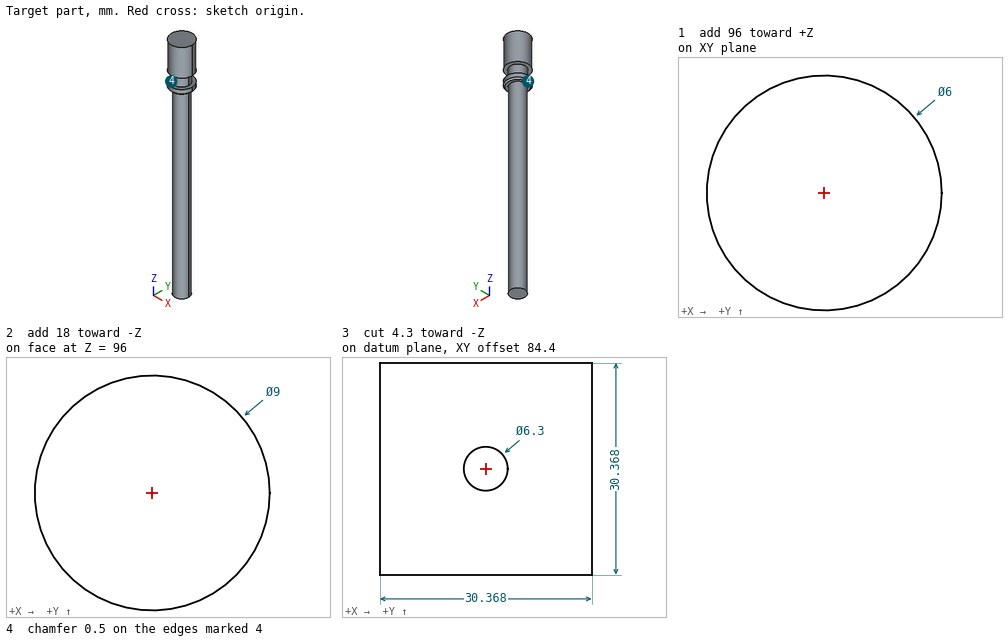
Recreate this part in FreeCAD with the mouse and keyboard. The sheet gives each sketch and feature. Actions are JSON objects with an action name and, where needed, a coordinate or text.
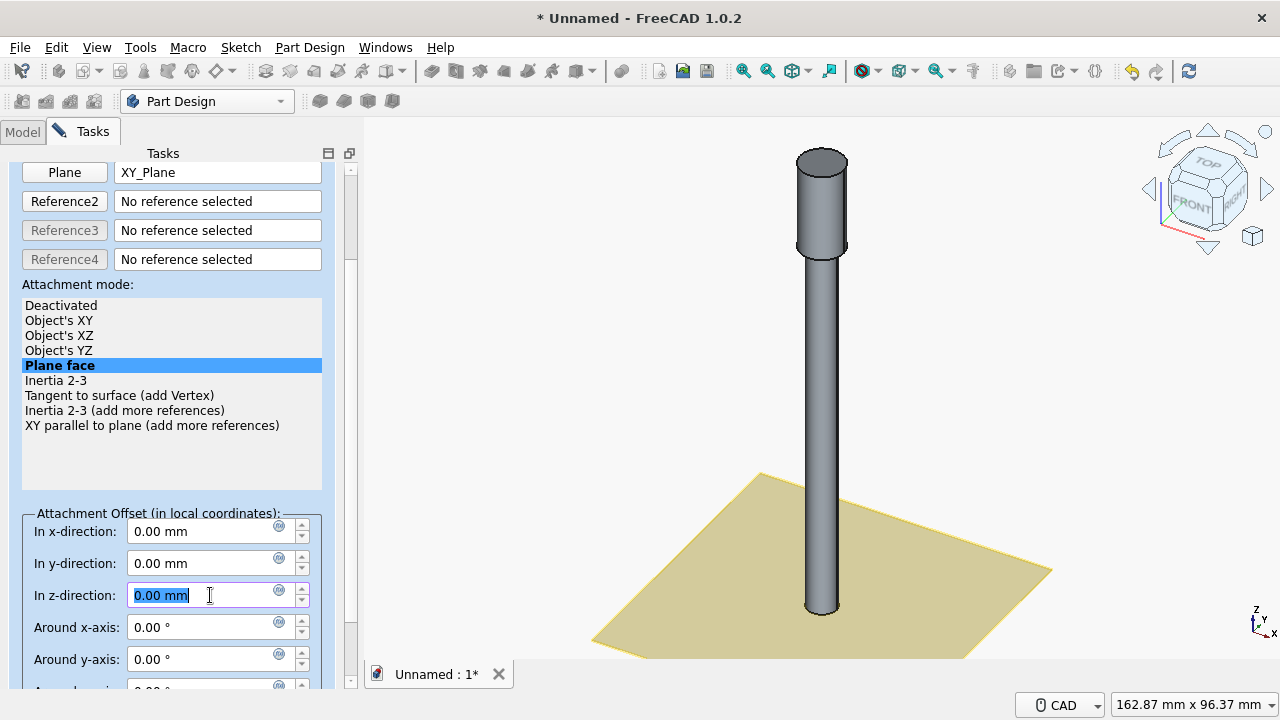
{"action": "type", "text": "84.4"}
{"action": "key", "text": "Tab"}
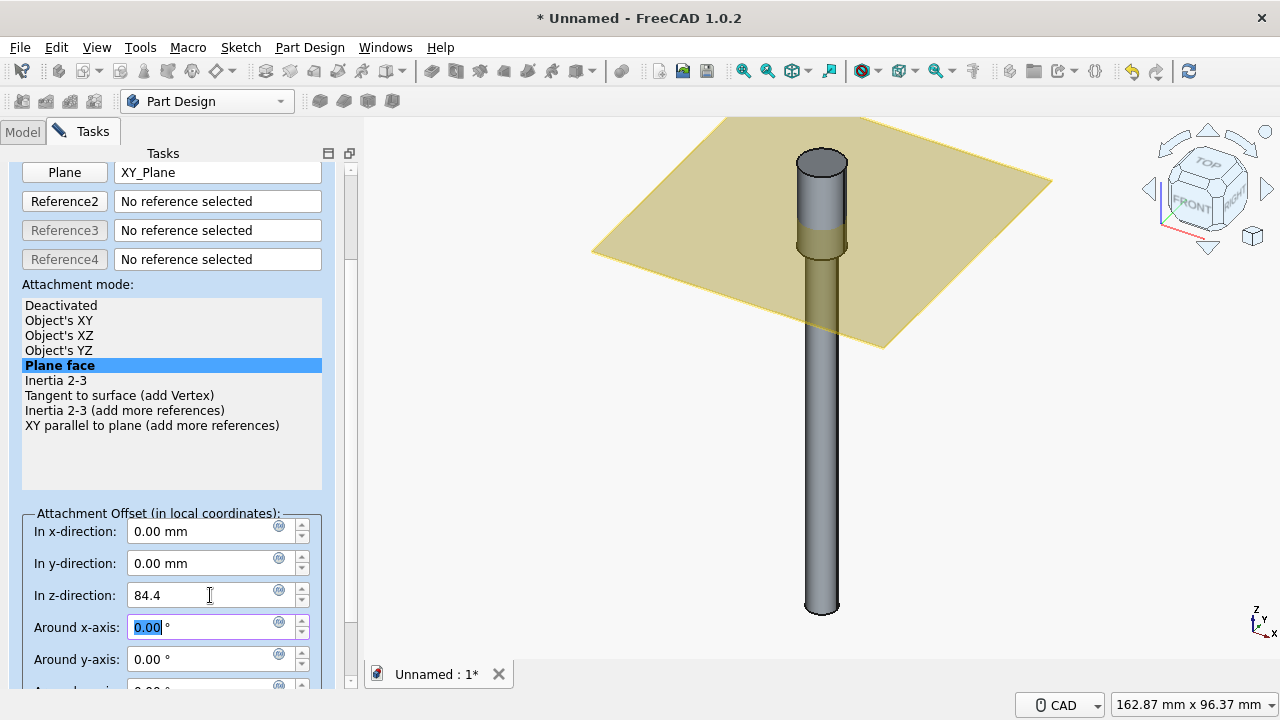
{"action": "scroll", "coordinate": [351, 426], "scroll_direction": "up", "scroll_amount": 3}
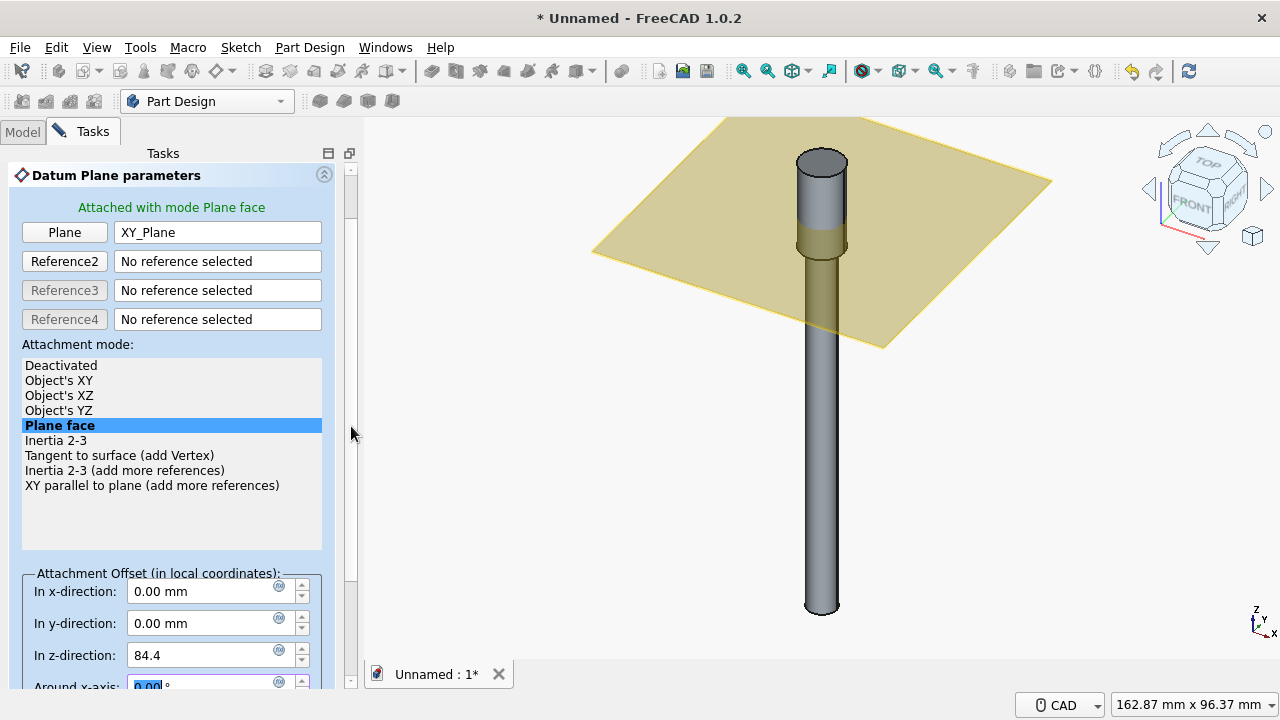
{"action": "left_click", "coordinate": [124, 192]}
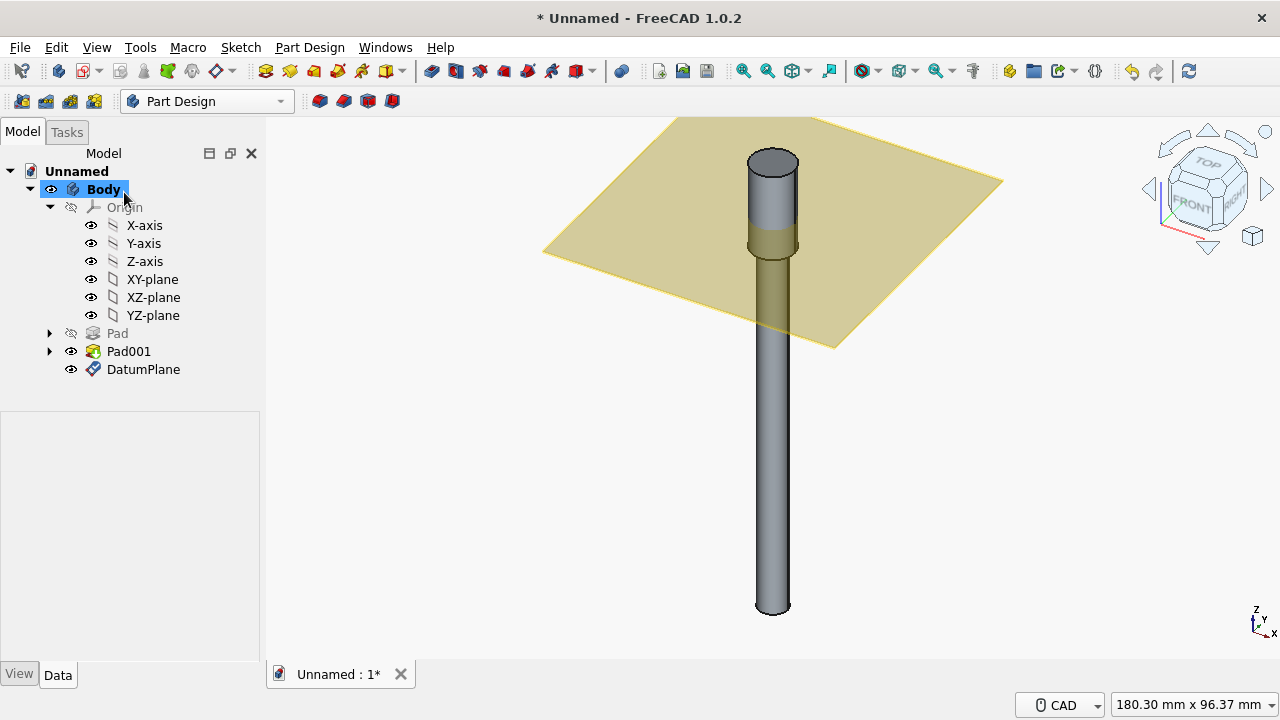
{"action": "left_click", "coordinate": [116, 369]}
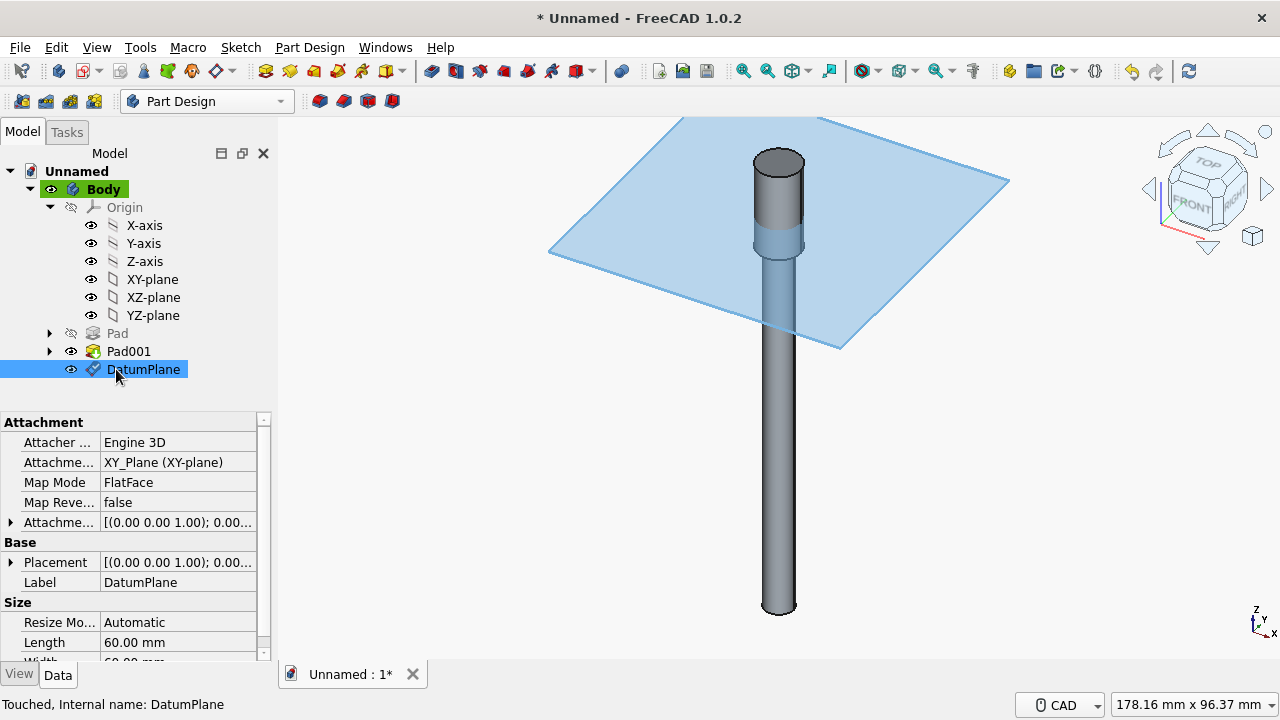
{"action": "left_click", "coordinate": [84, 72]}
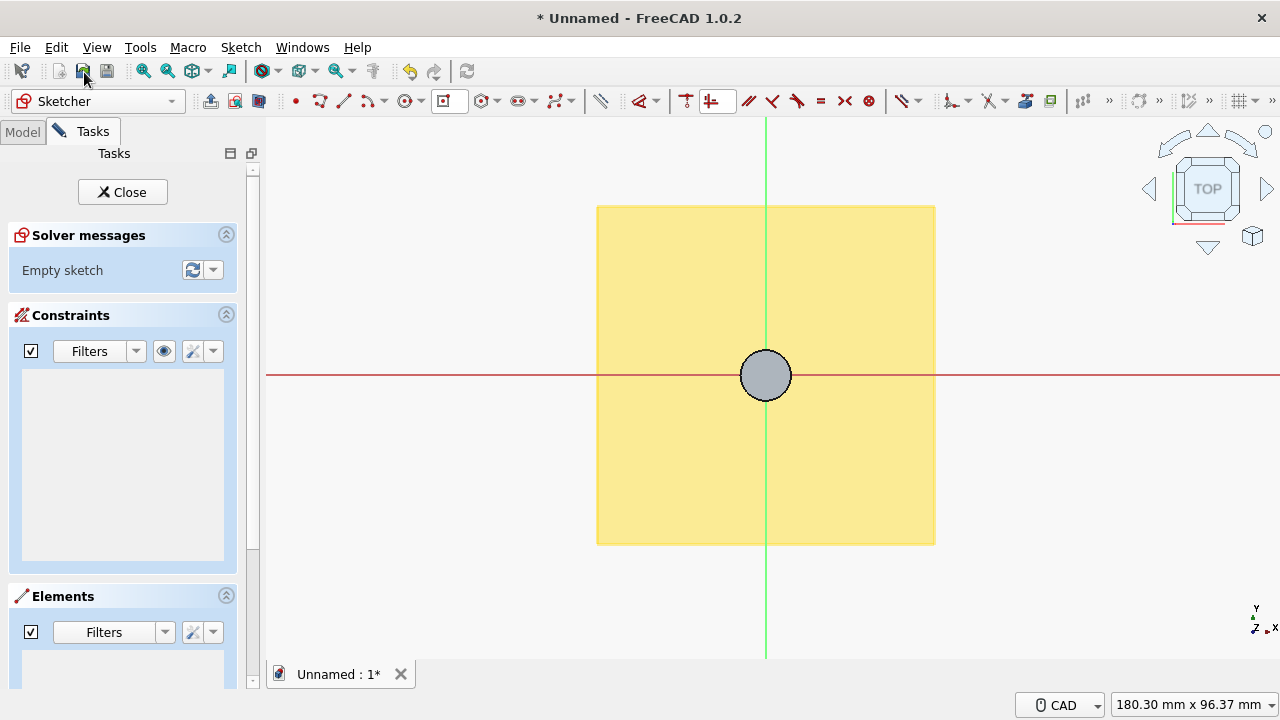
{"action": "left_click", "coordinate": [260, 102]}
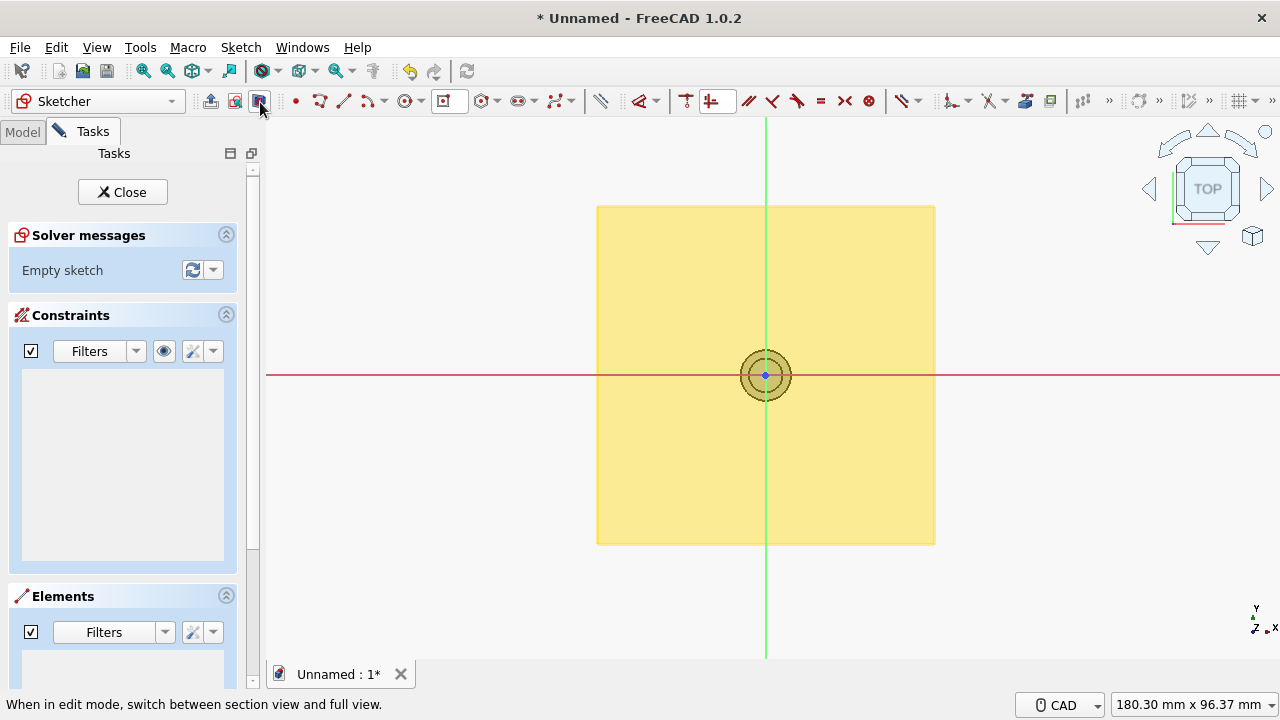
{"action": "scroll", "coordinate": [840, 360], "scroll_direction": "up", "scroll_amount": 3}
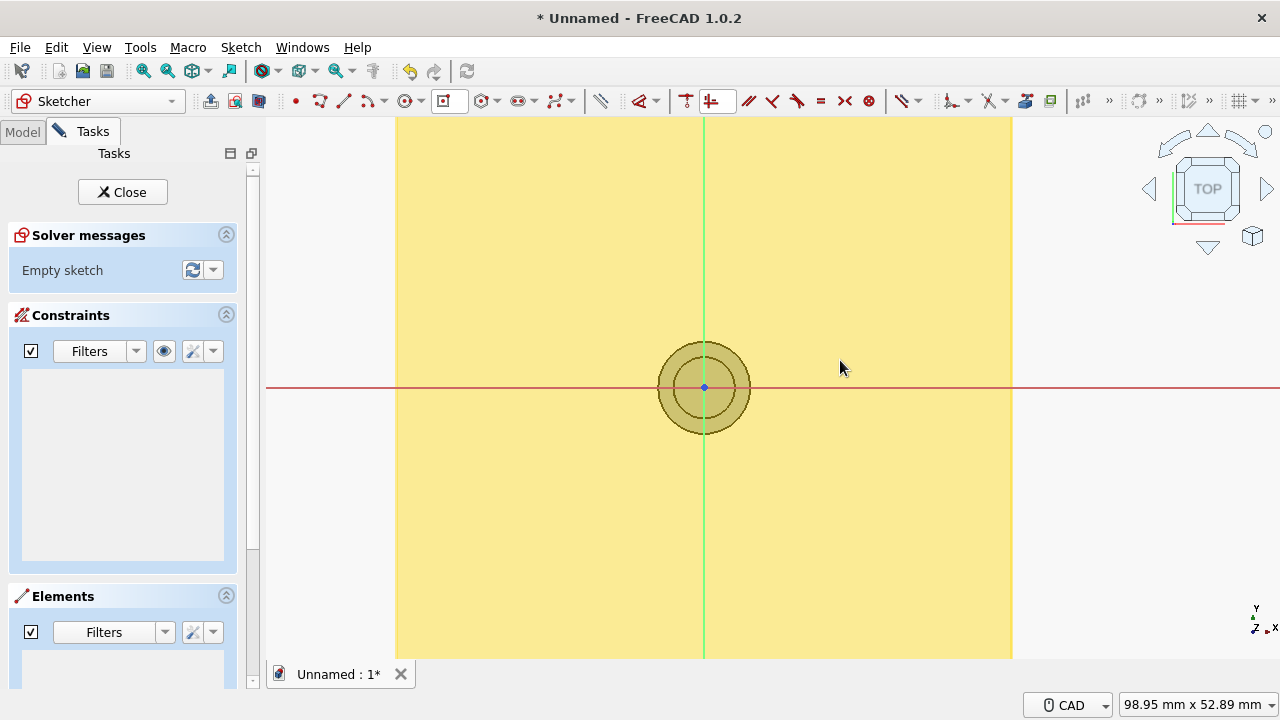
{"action": "key", "text": "g v"}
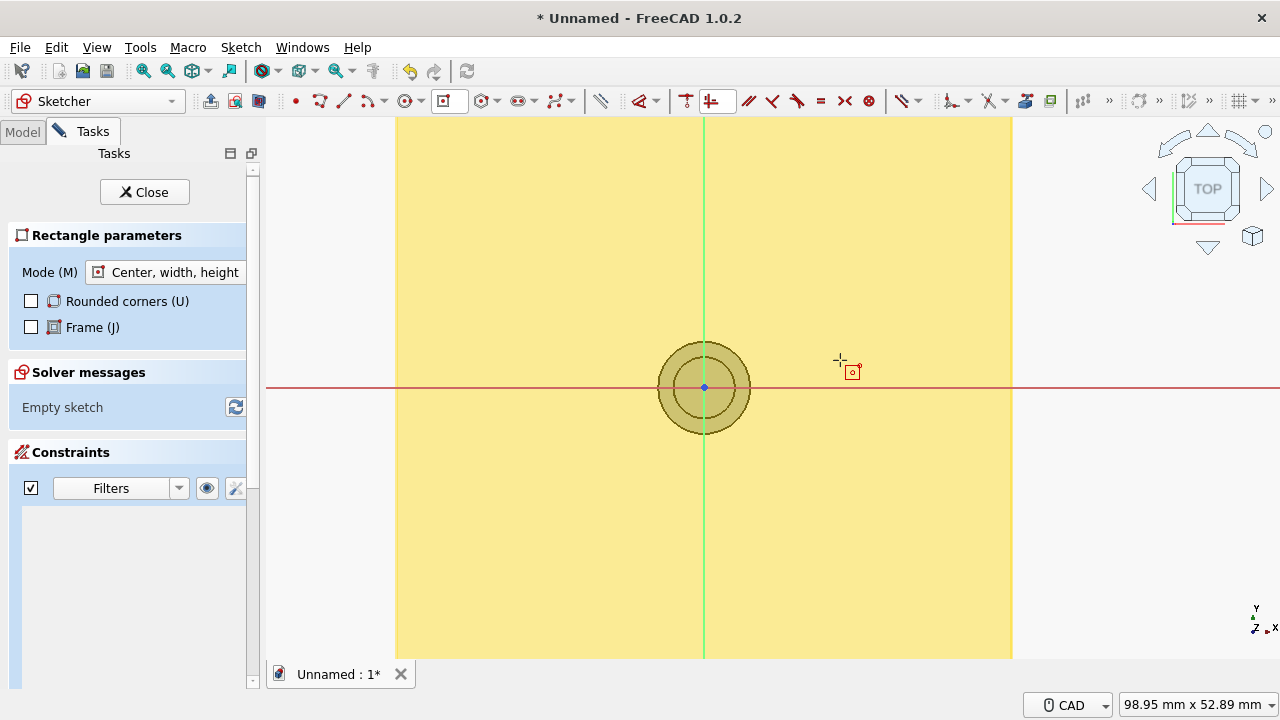
{"action": "left_click", "coordinate": [704, 388]}
{"action": "left_click", "coordinate": [860, 232]}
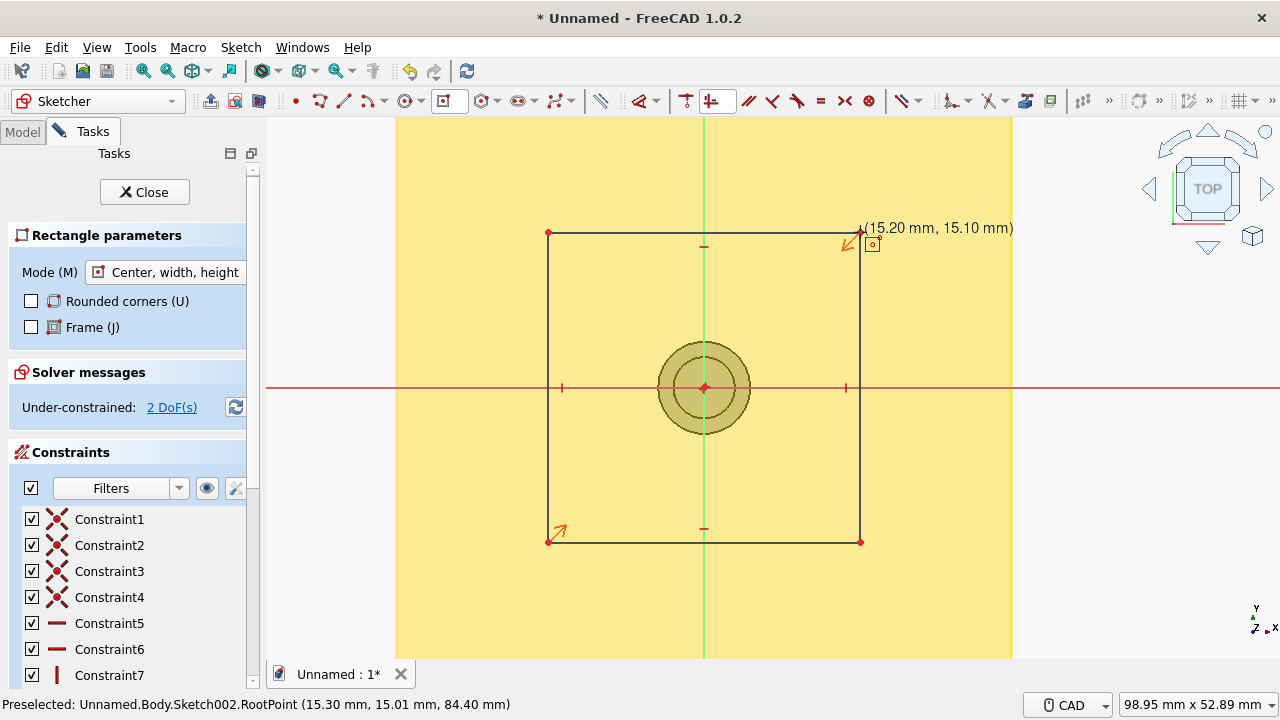
{"action": "key", "text": "g c"}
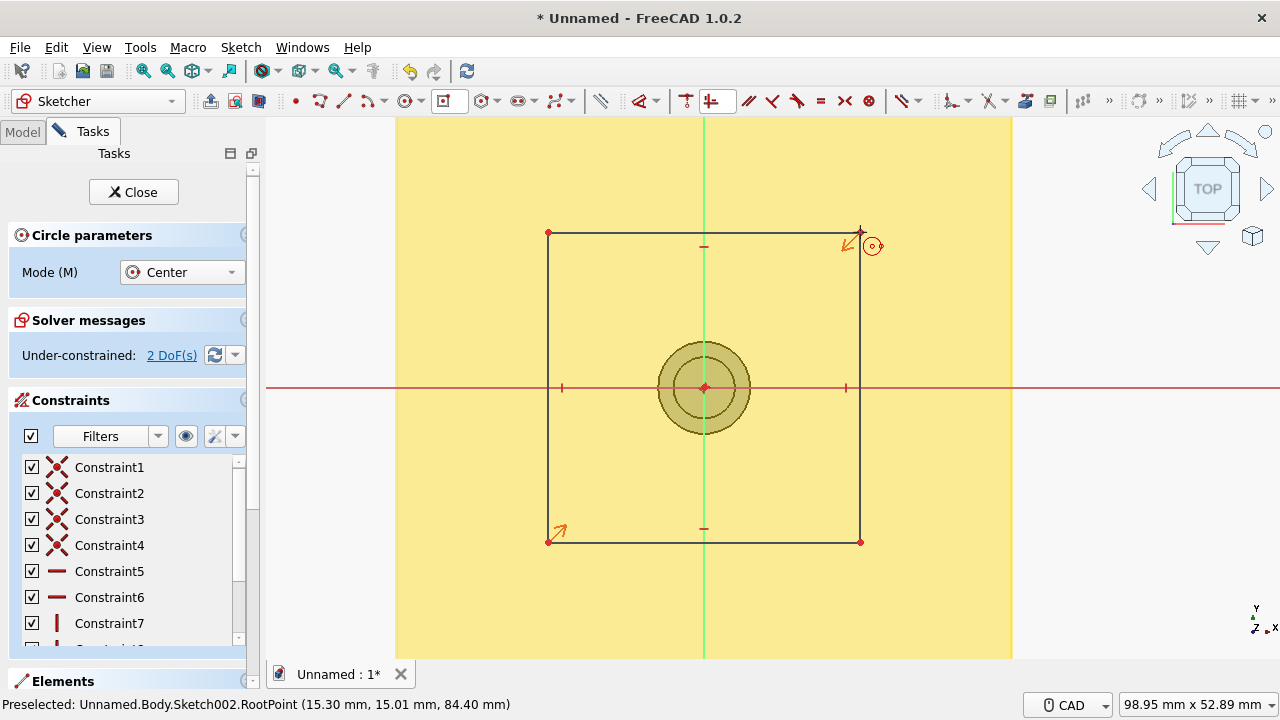
{"action": "left_click", "coordinate": [704, 388]}
{"action": "left_click", "coordinate": [727, 365]}
{"action": "key", "text": "Escape"}